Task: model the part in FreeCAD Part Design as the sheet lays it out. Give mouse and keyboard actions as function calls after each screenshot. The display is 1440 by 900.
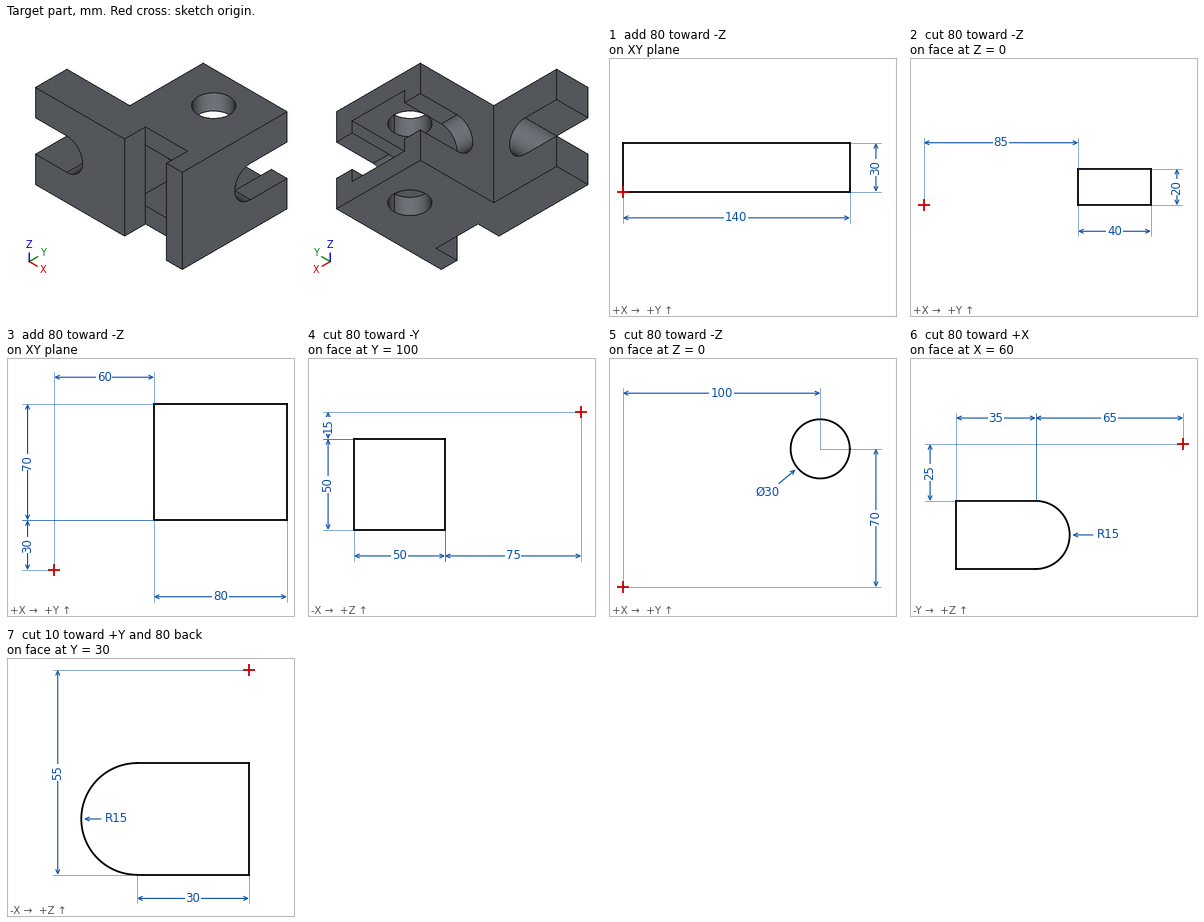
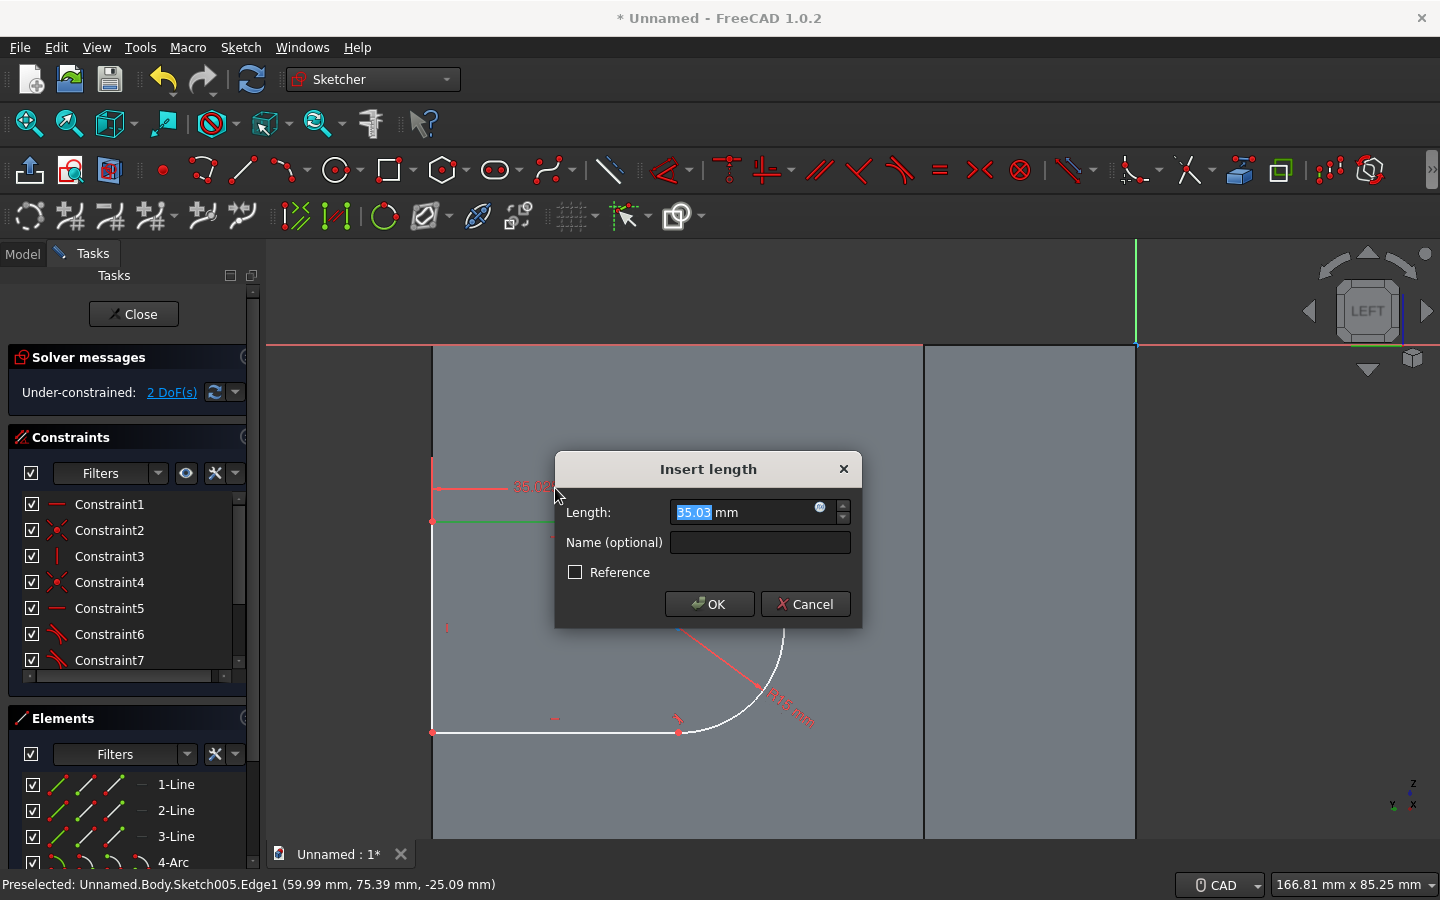
text(35)
key(Return)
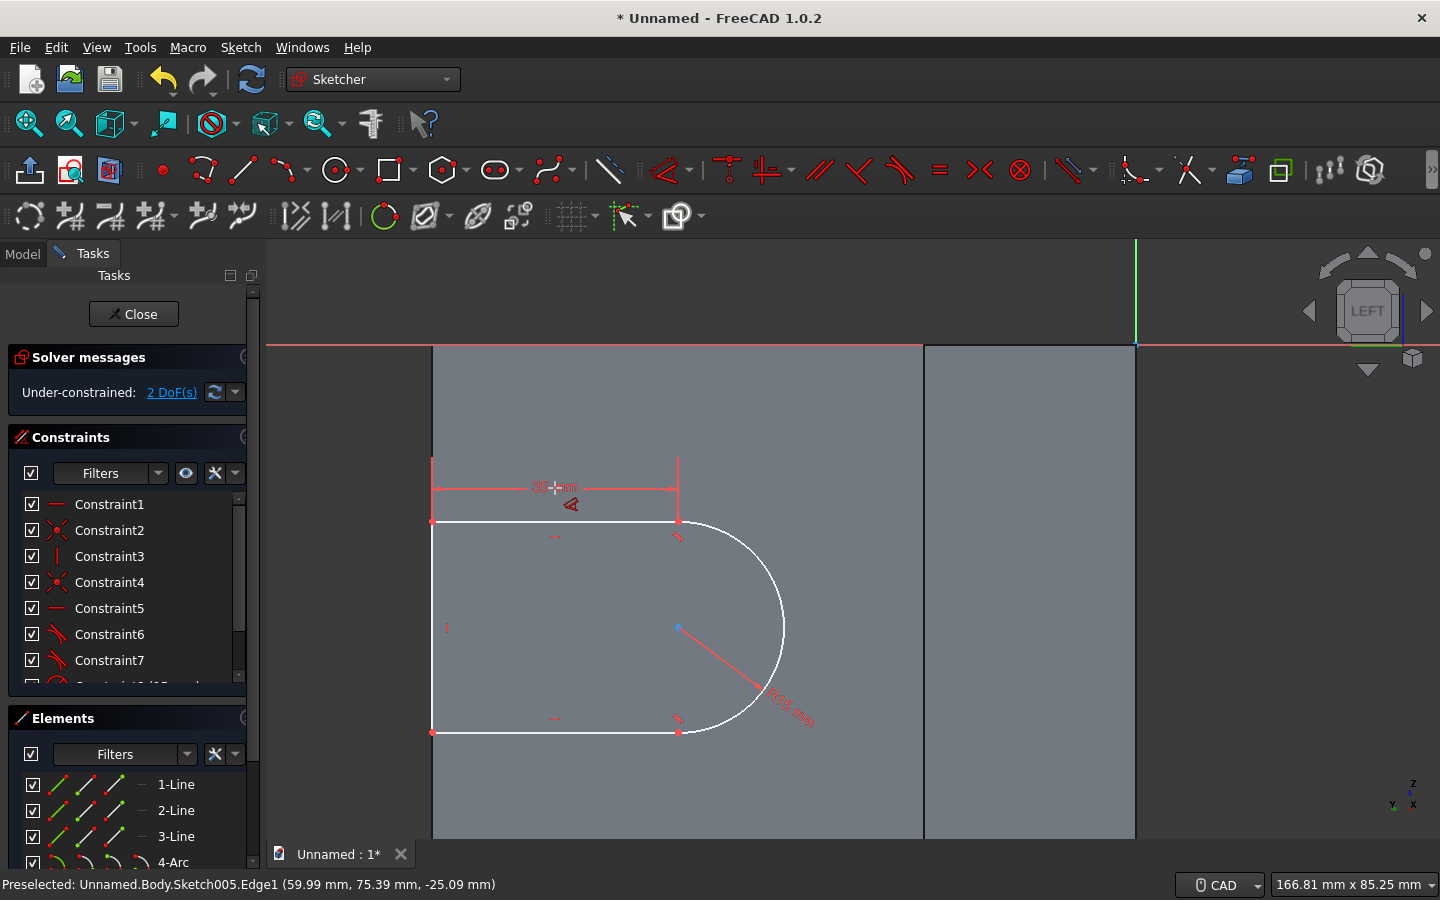
click(678, 522)
click(907, 311)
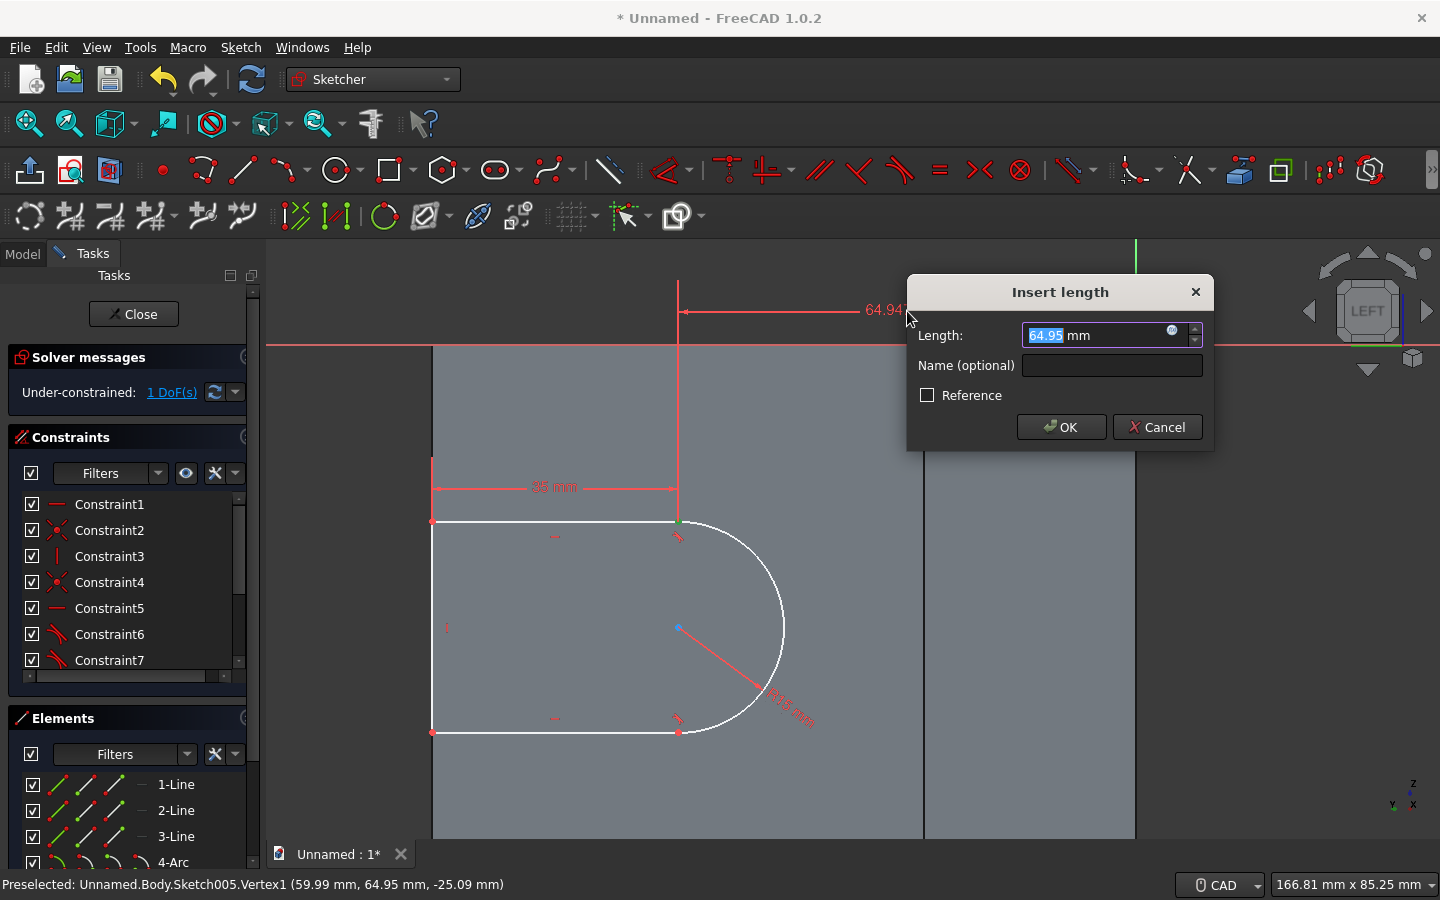
text(65)
key(Return)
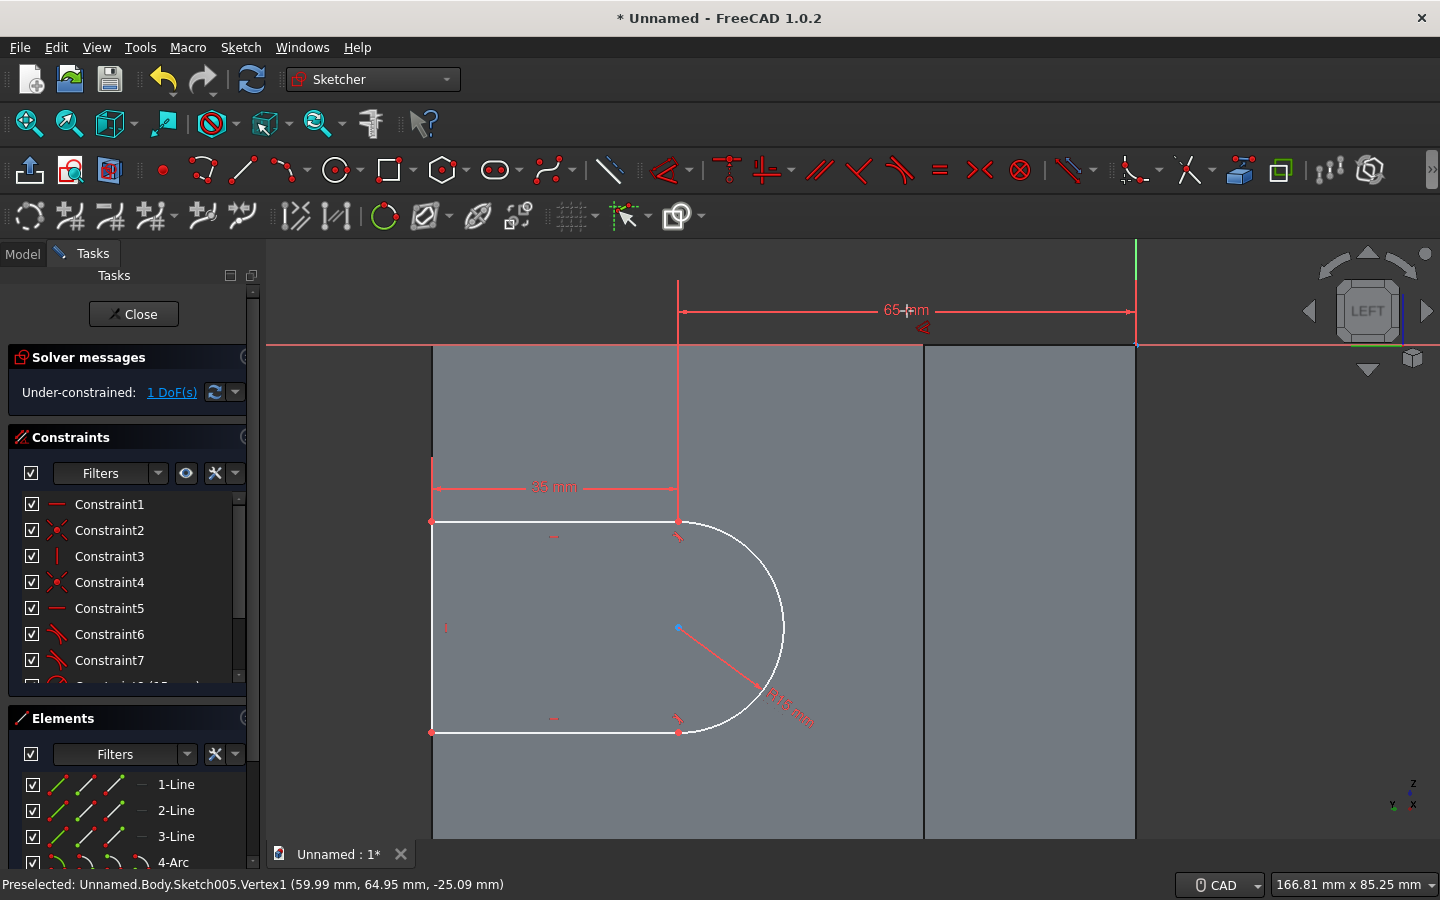
click(678, 522)
click(1170, 434)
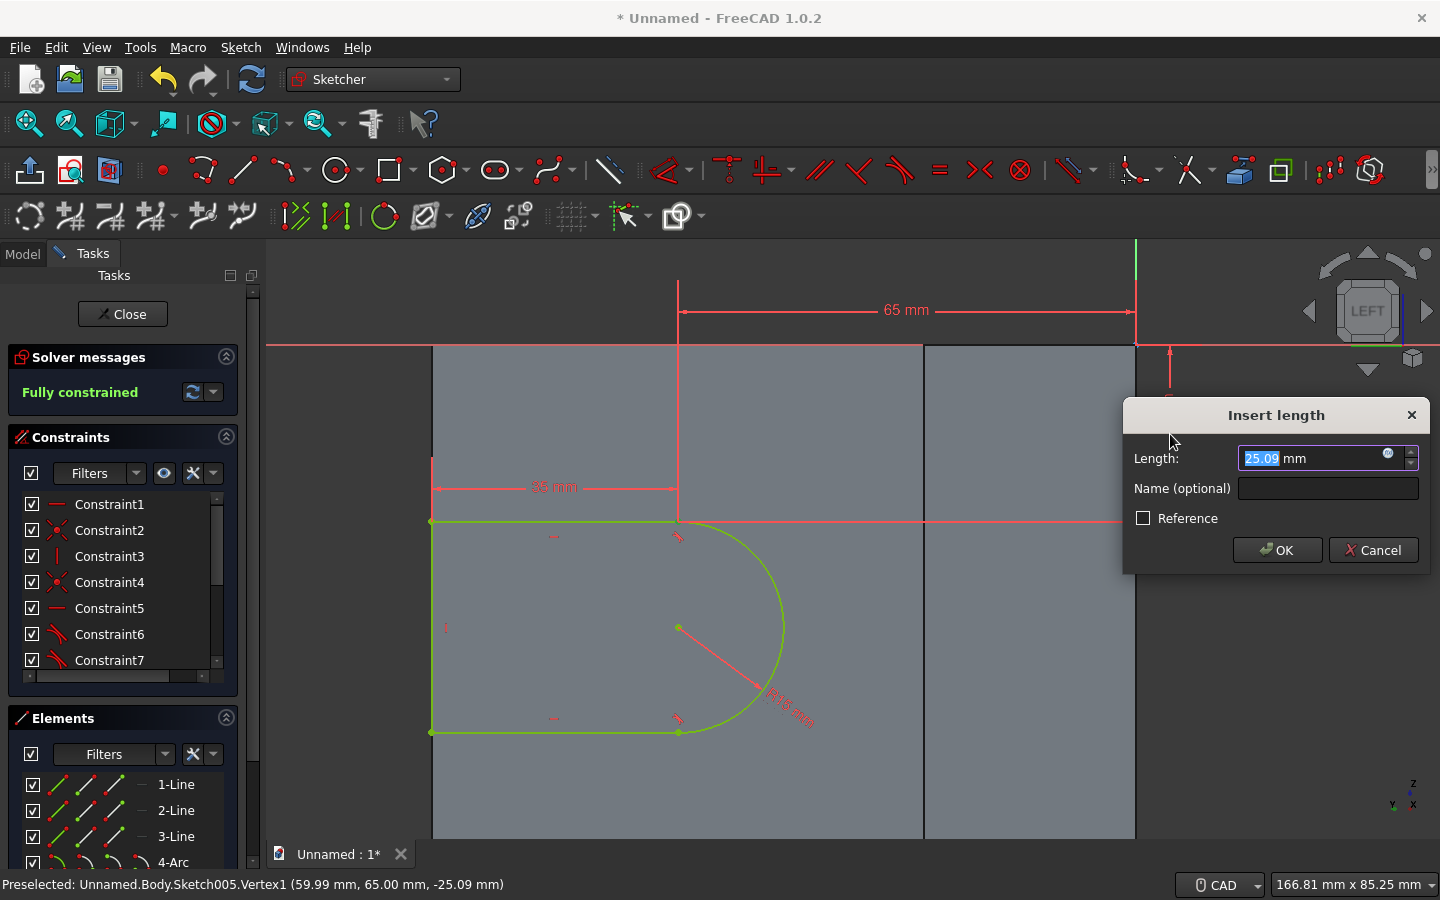
text(25)
key(Return)
key(Escape)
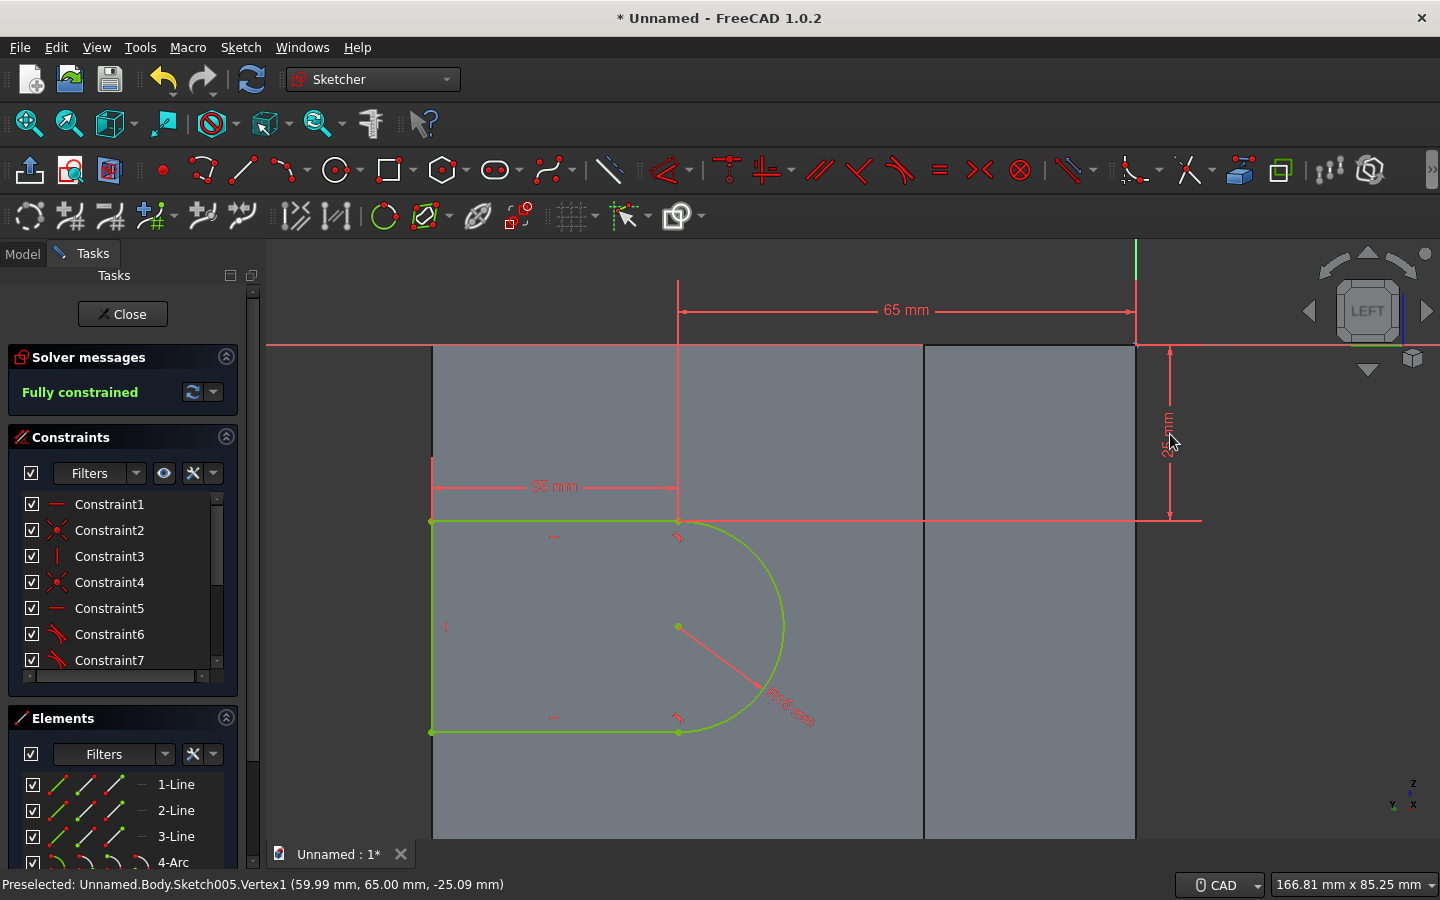
click(123, 314)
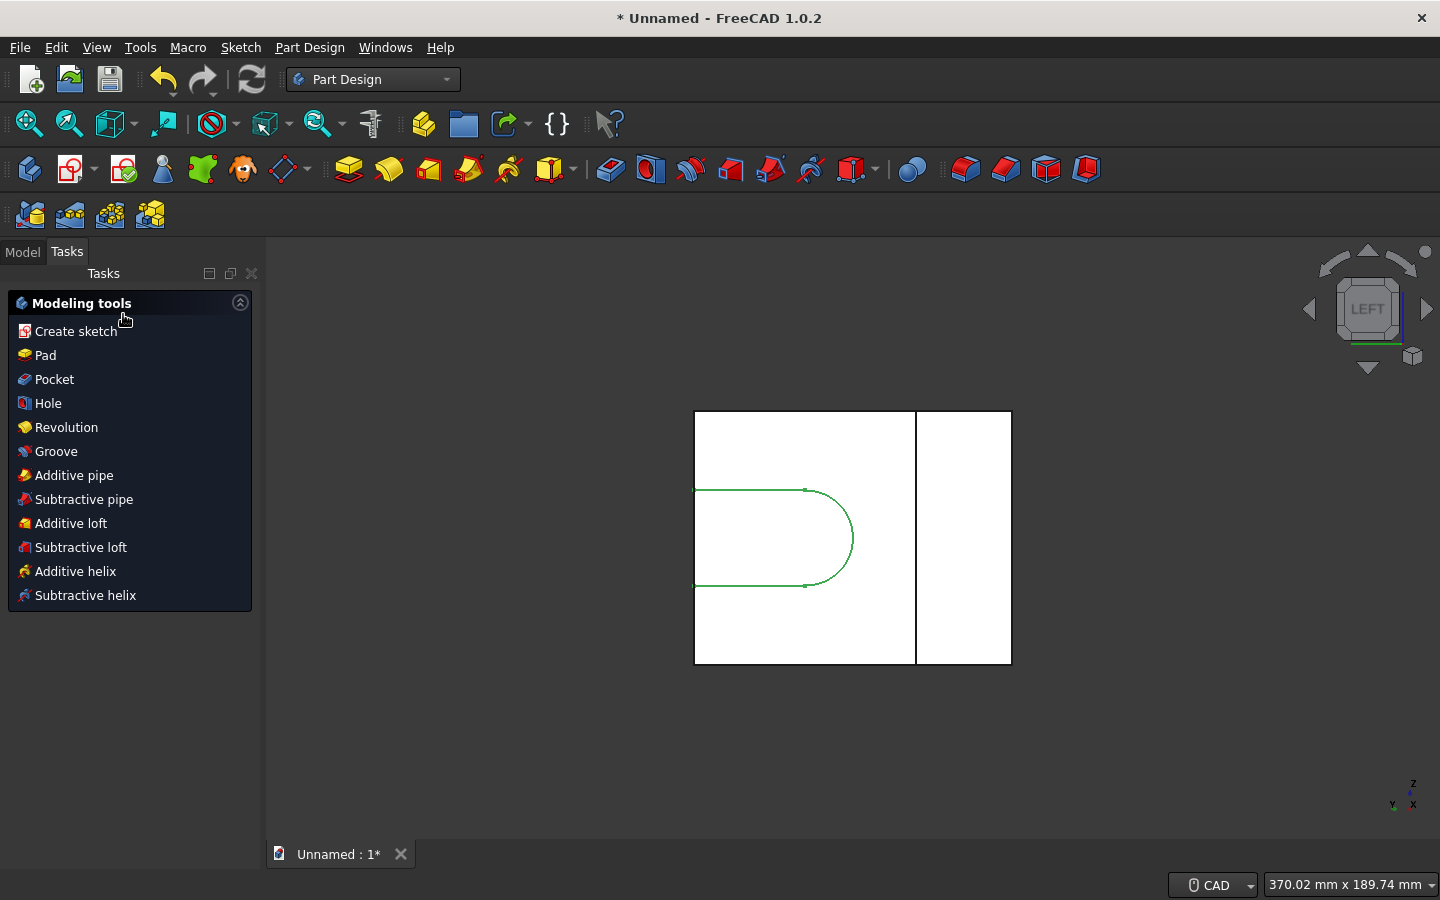
click(612, 170)